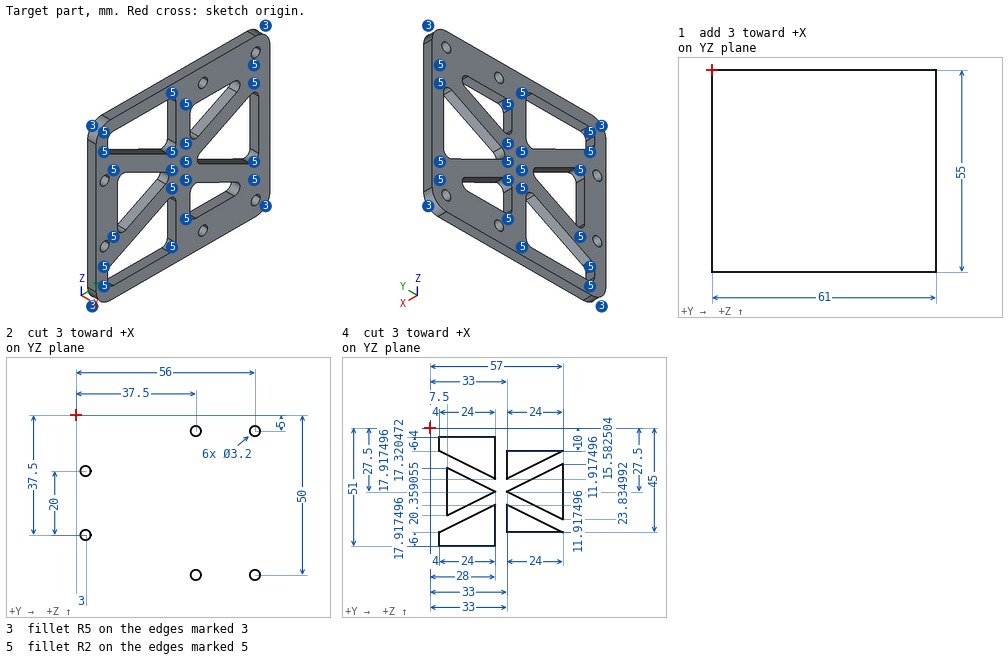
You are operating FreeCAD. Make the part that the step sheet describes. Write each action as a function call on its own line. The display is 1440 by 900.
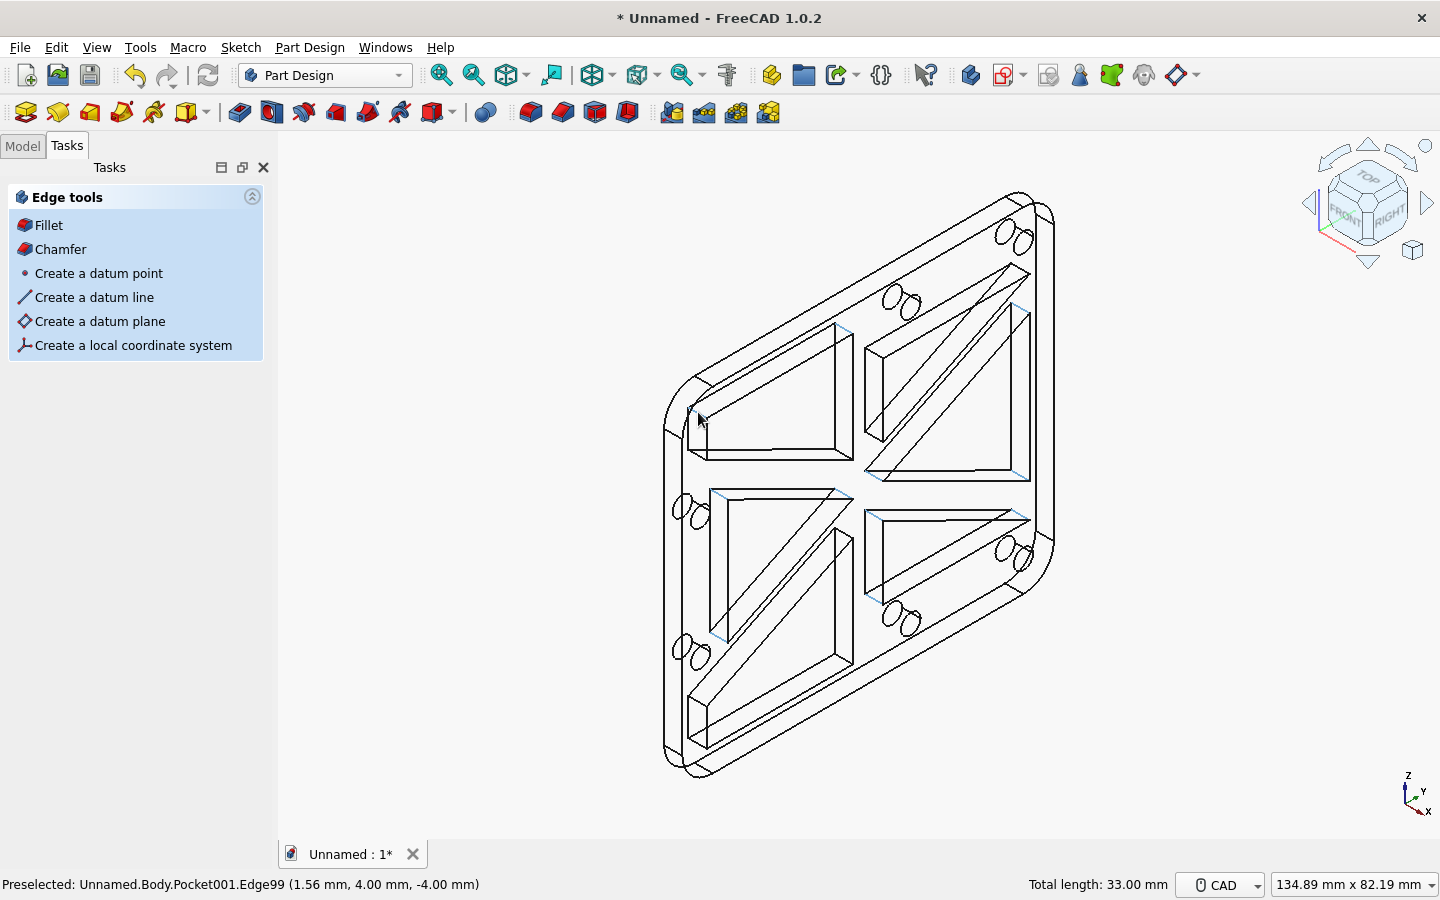
click(698, 454, ctrl)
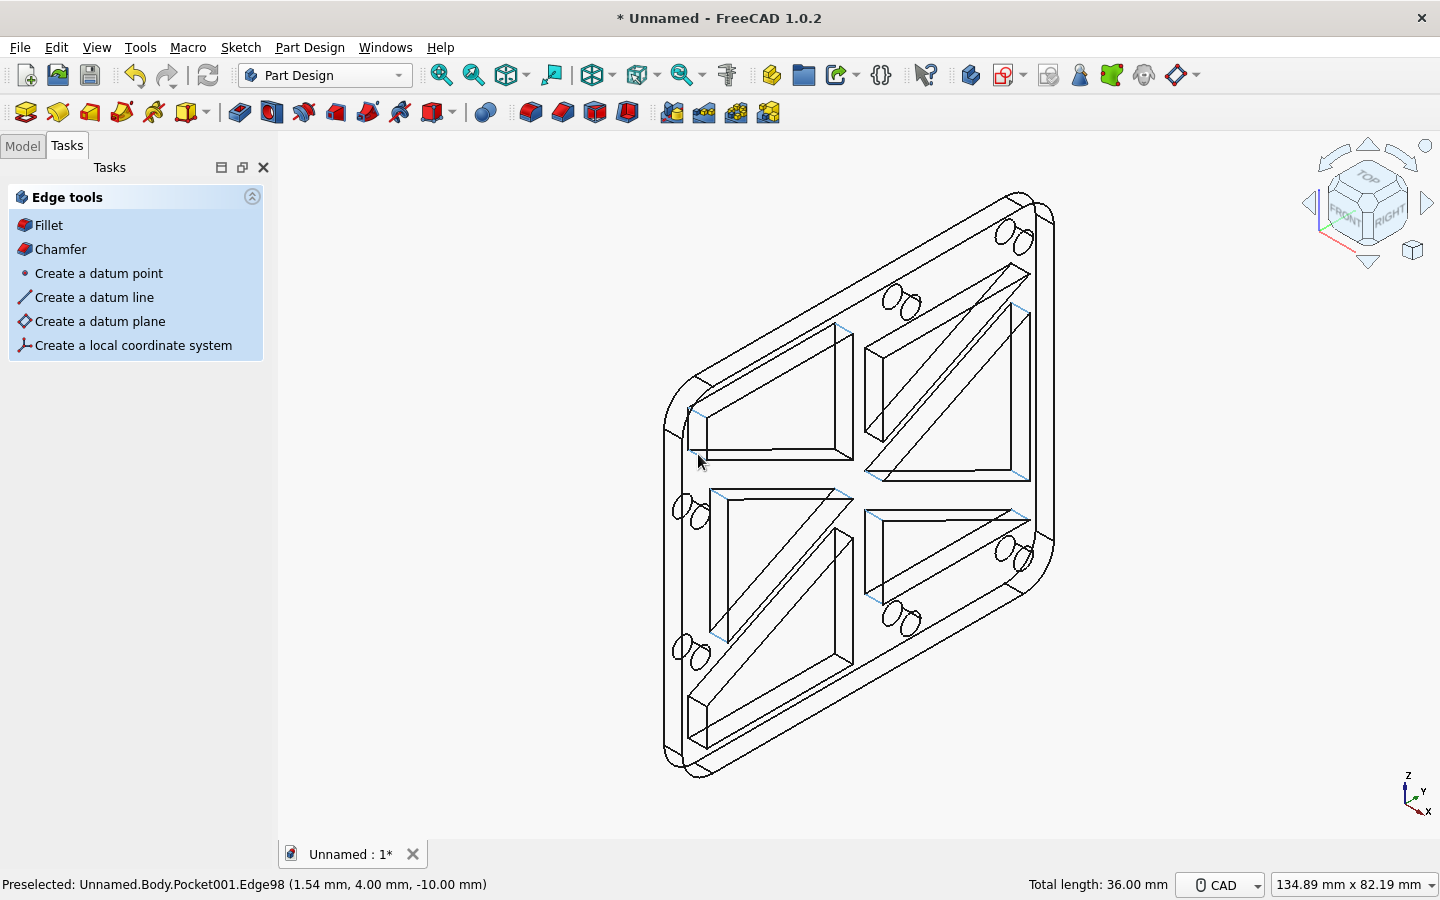
click(842, 452, ctrl)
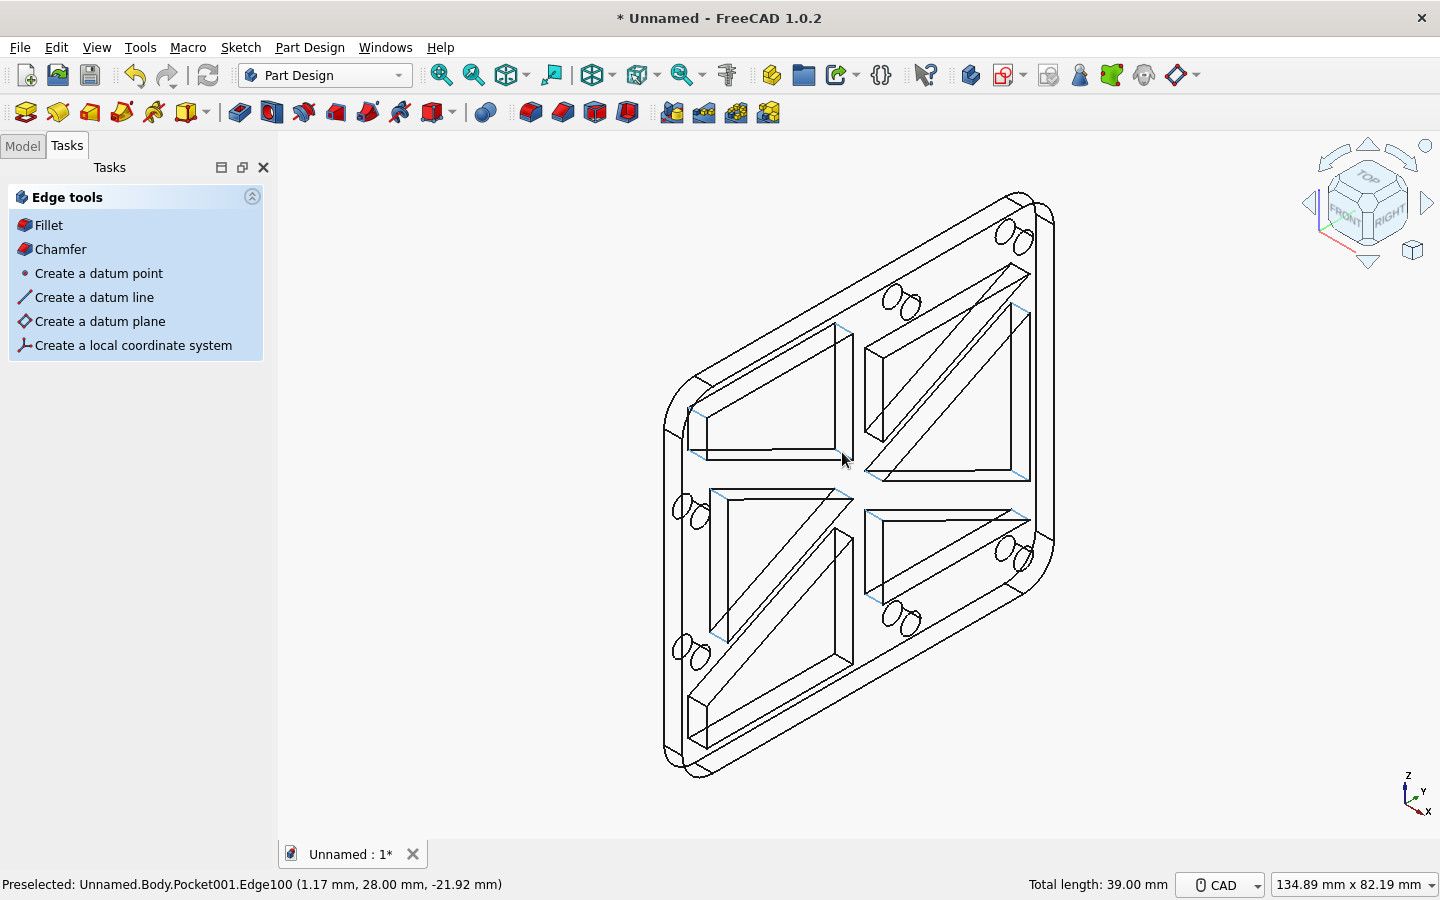
click(698, 742, ctrl)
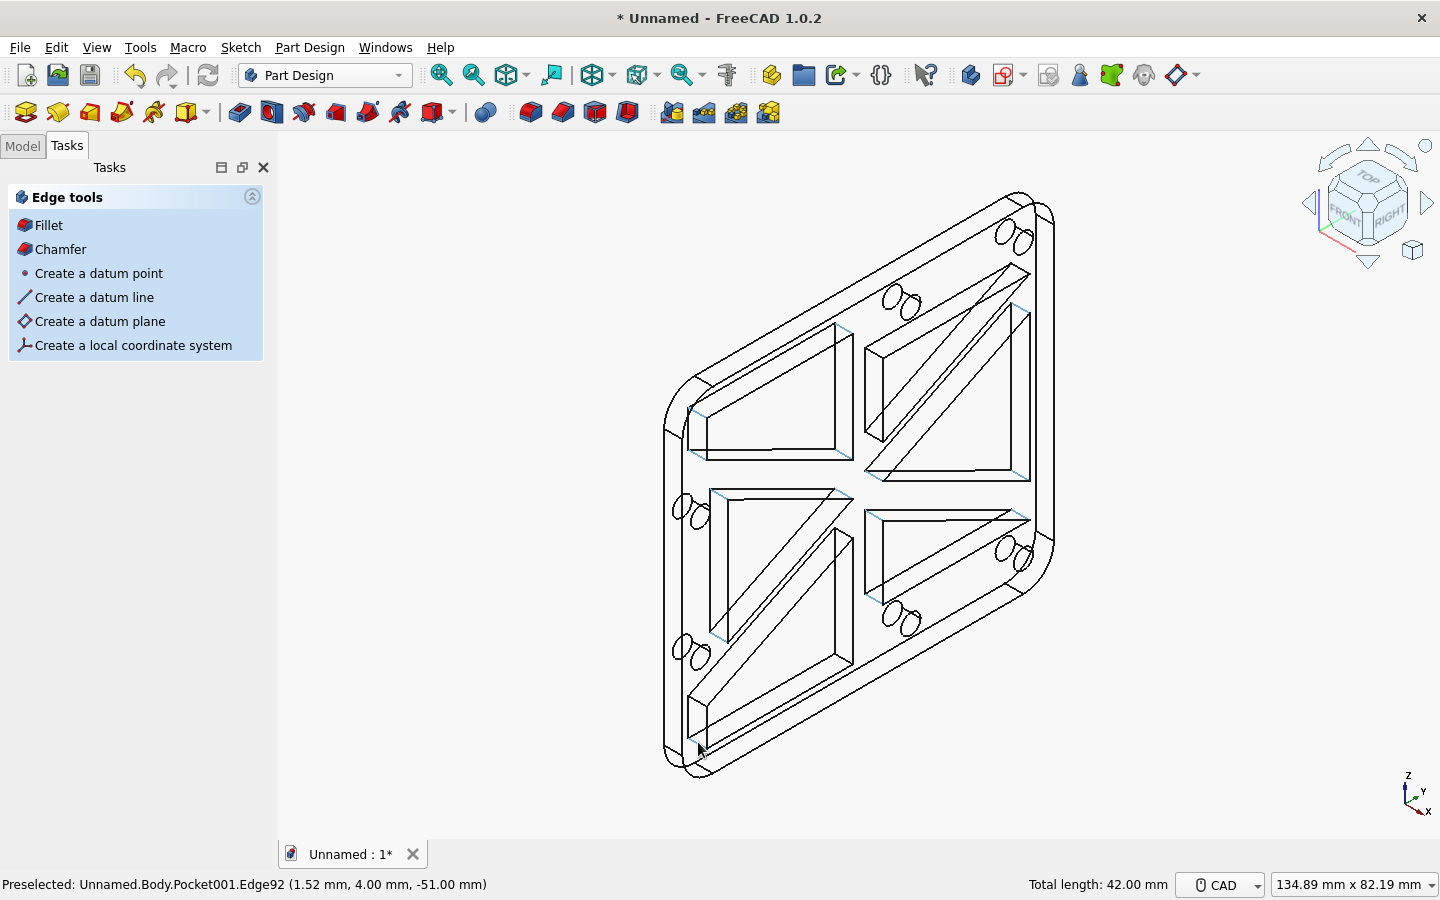
click(844, 658, ctrl)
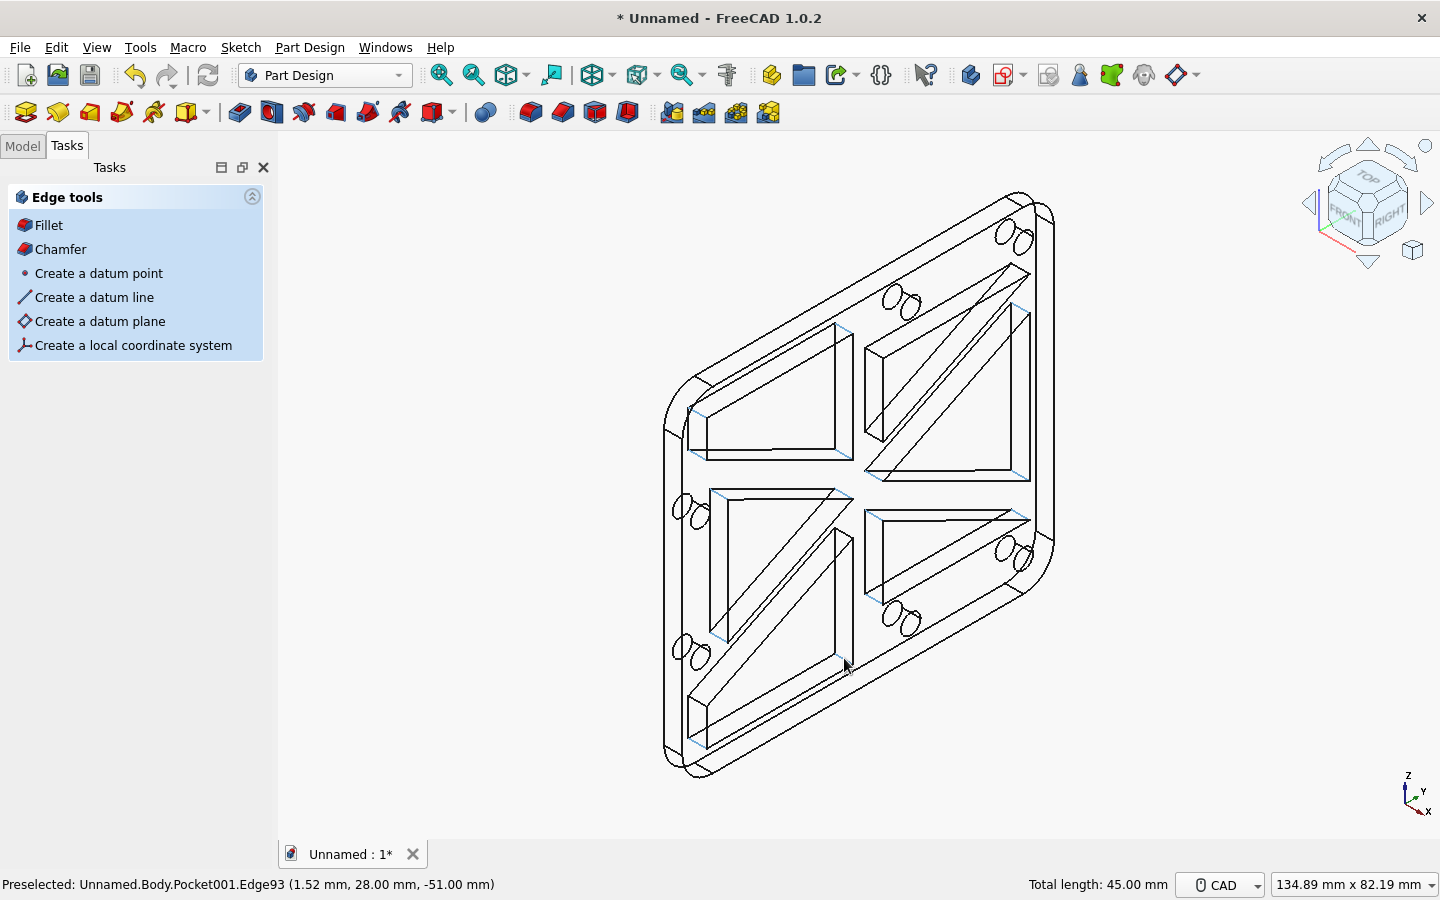
click(844, 532, ctrl)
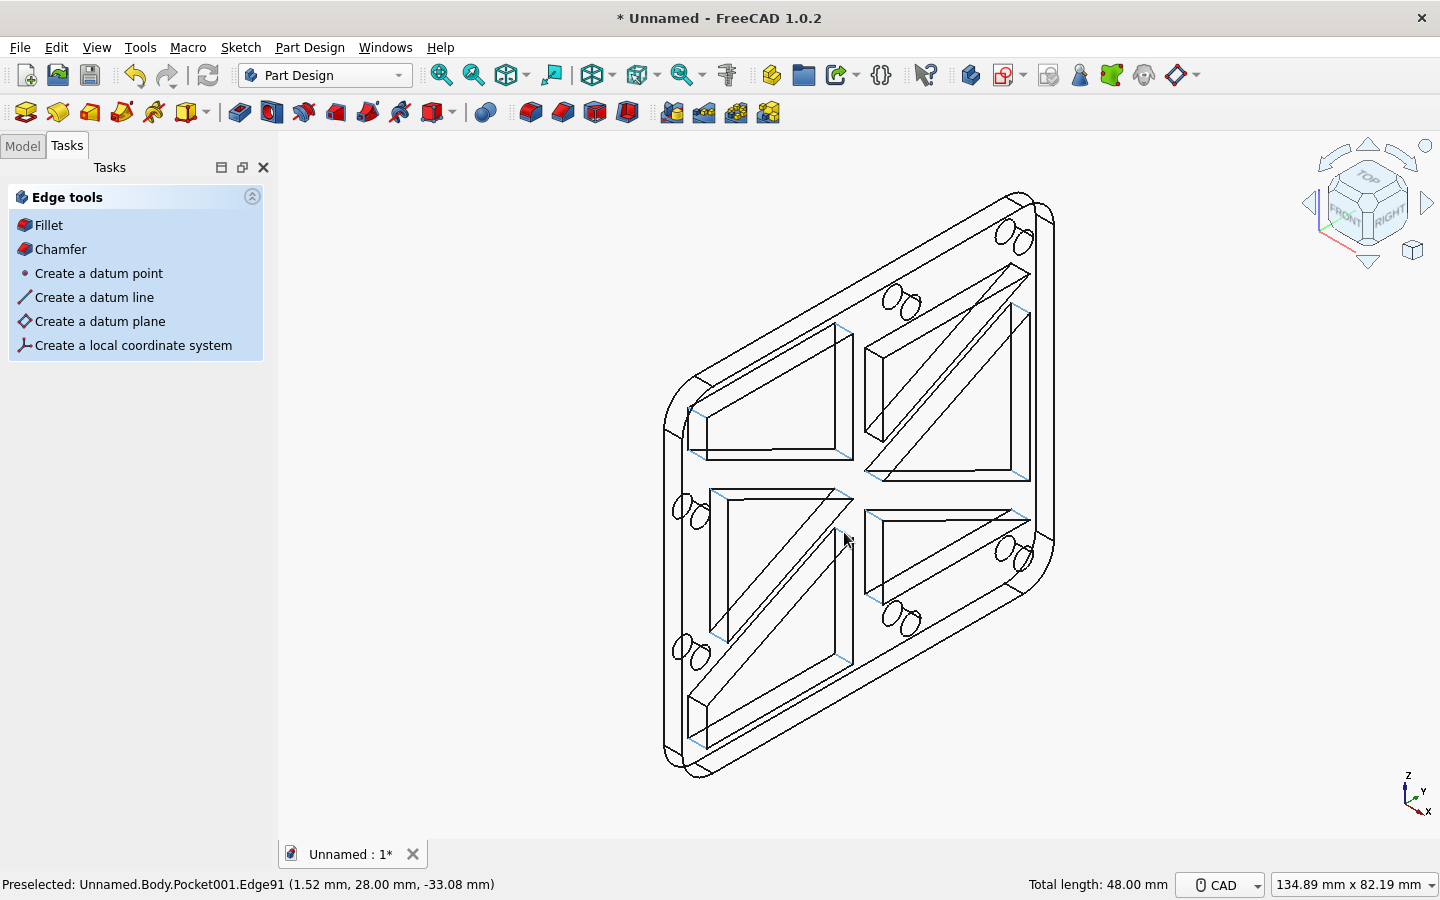
click(698, 700, ctrl)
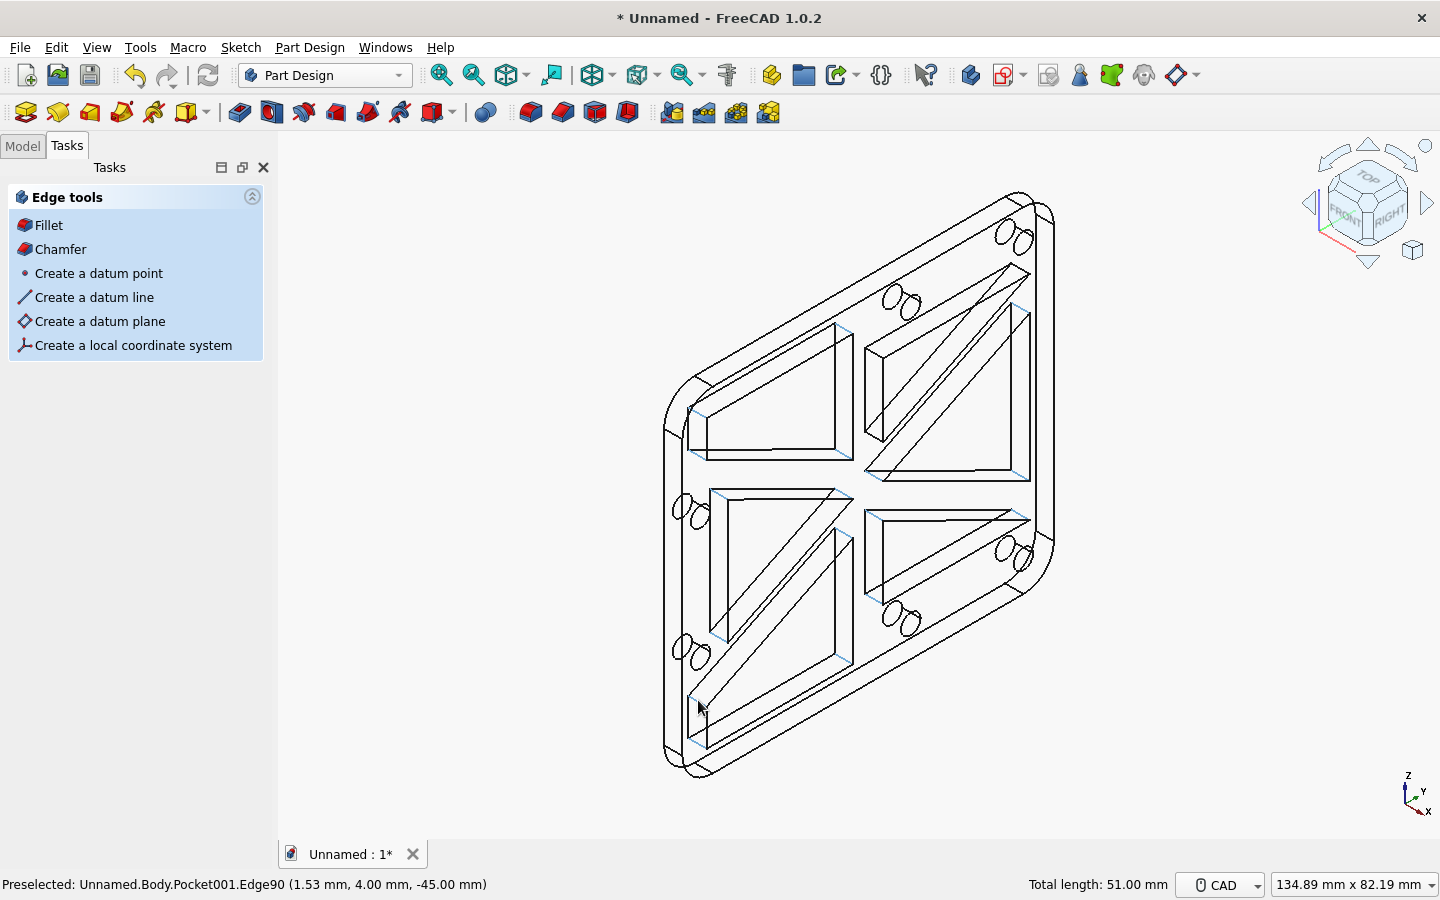
click(874, 352, ctrl)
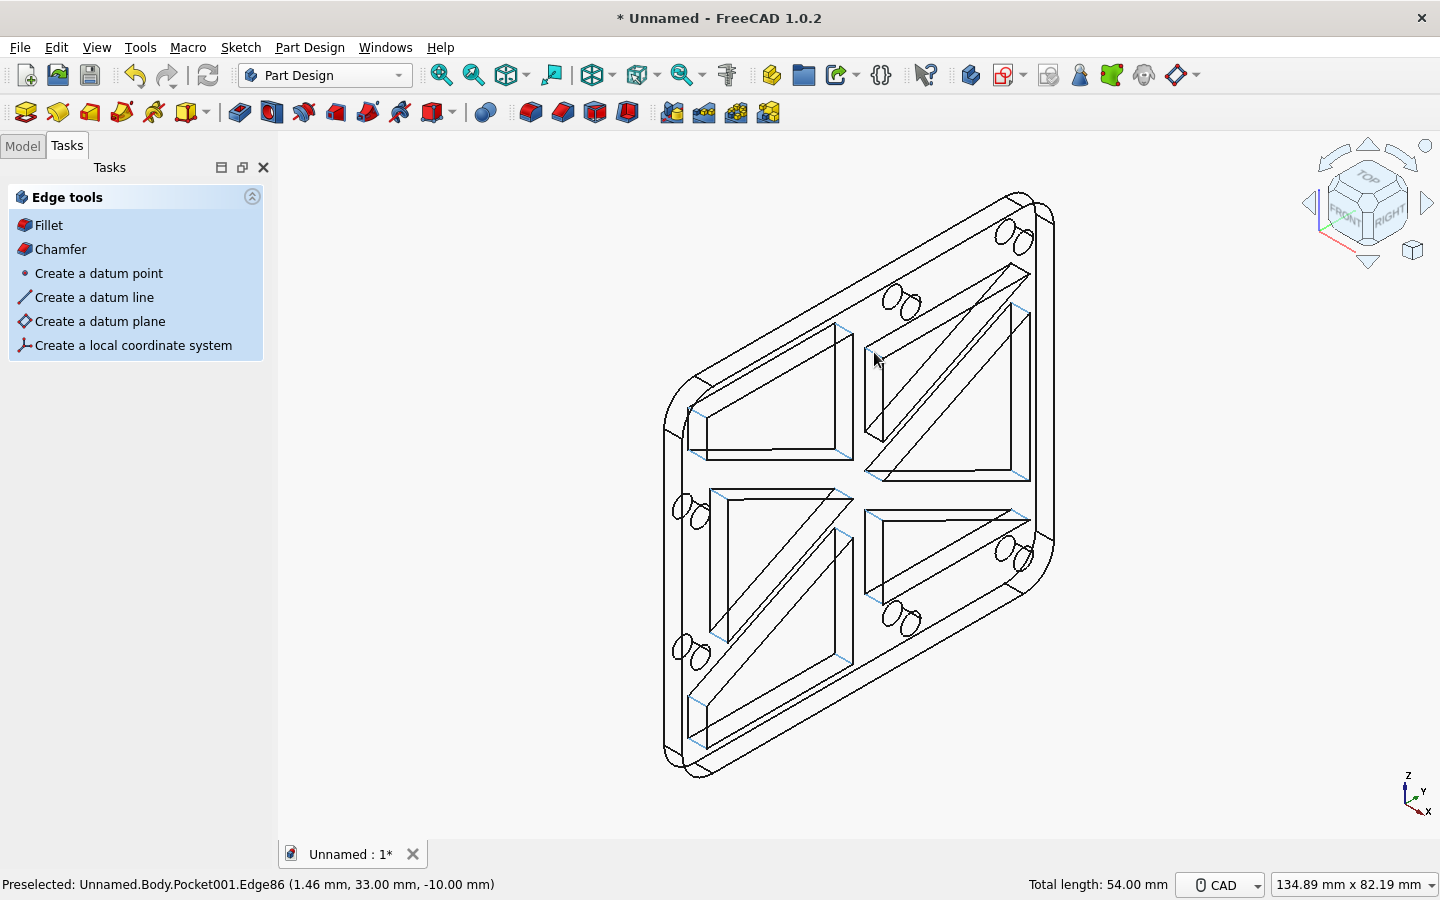
click(874, 436, ctrl)